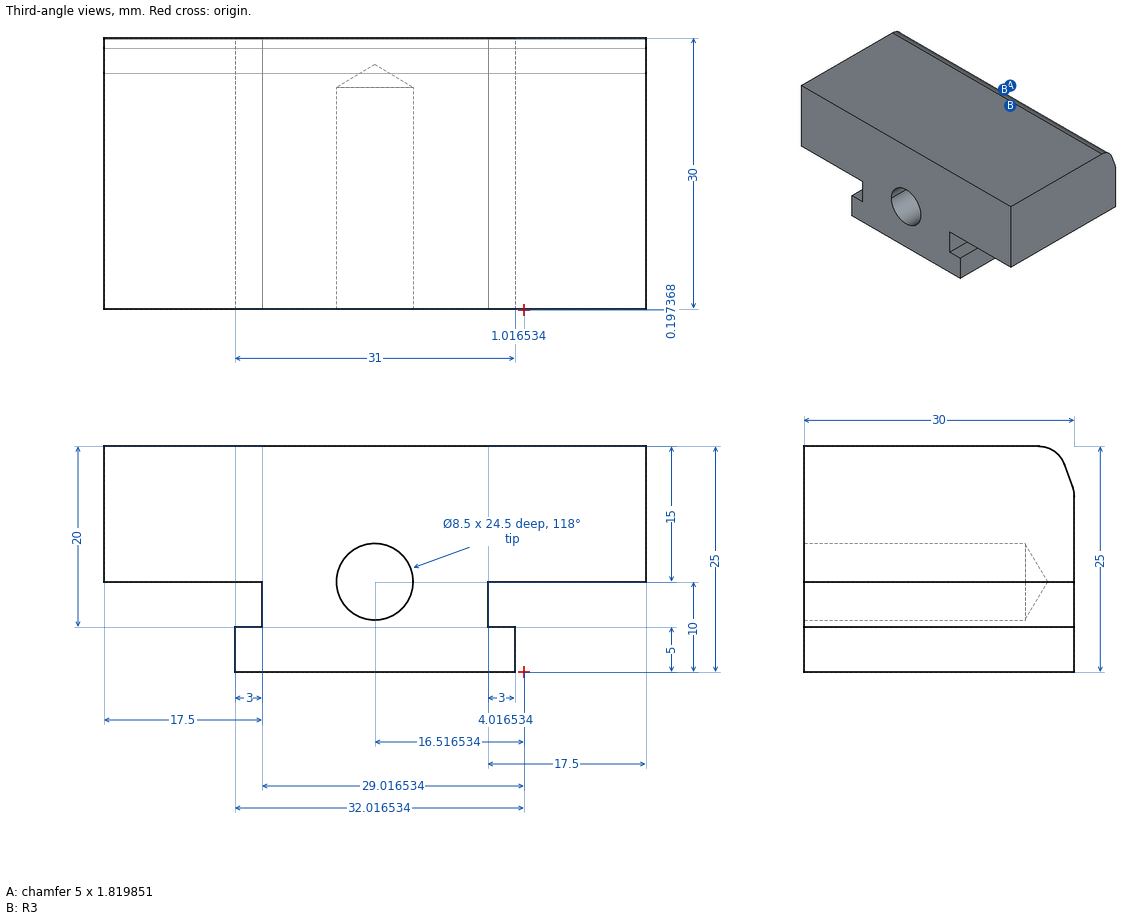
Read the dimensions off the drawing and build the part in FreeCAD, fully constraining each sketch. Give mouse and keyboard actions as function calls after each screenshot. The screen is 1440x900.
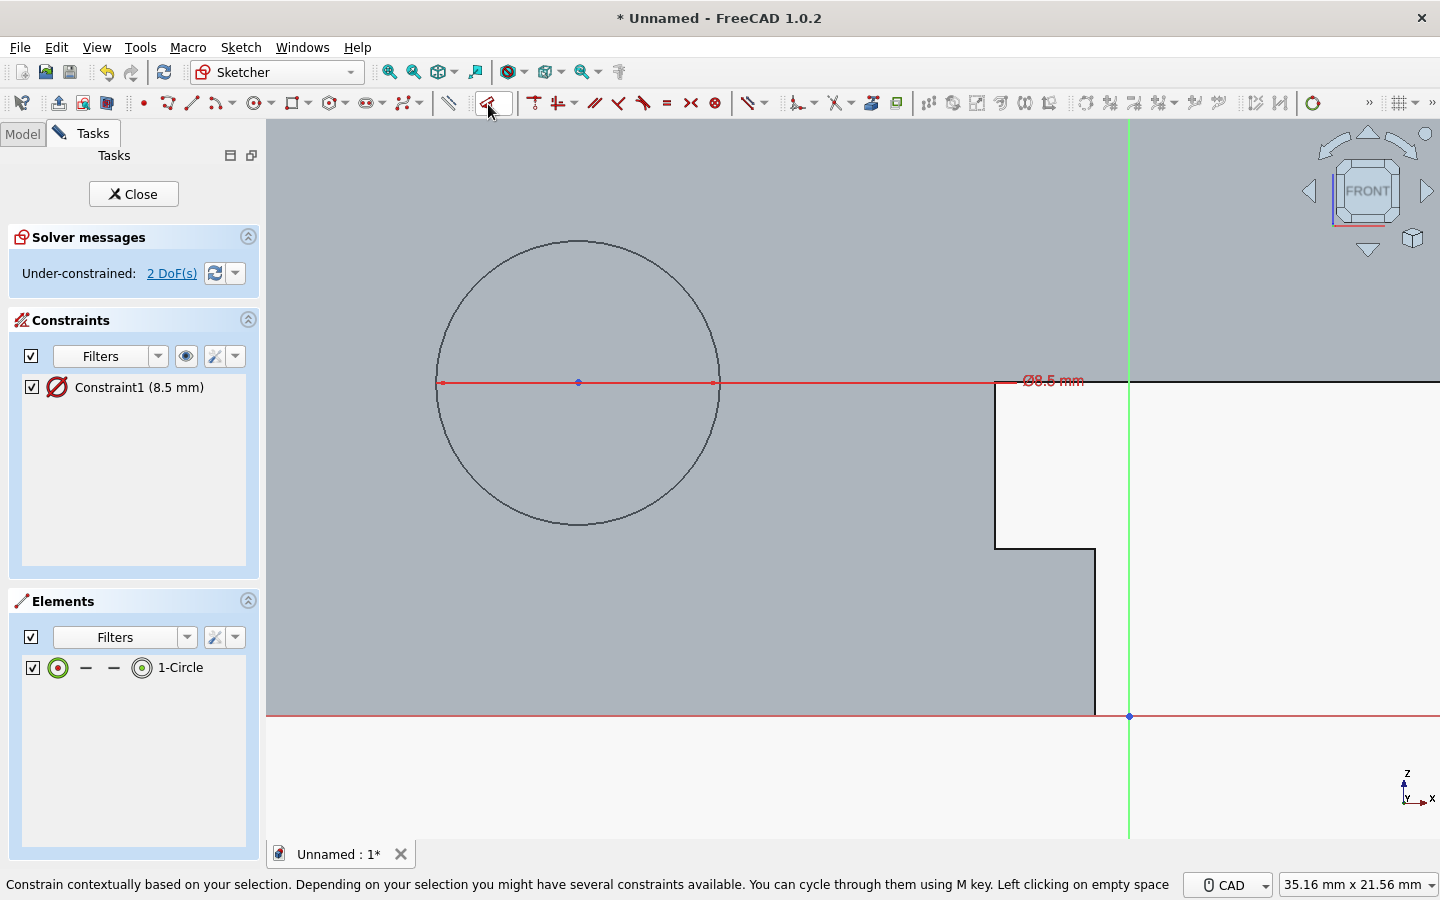
click(578, 383)
click(1163, 550)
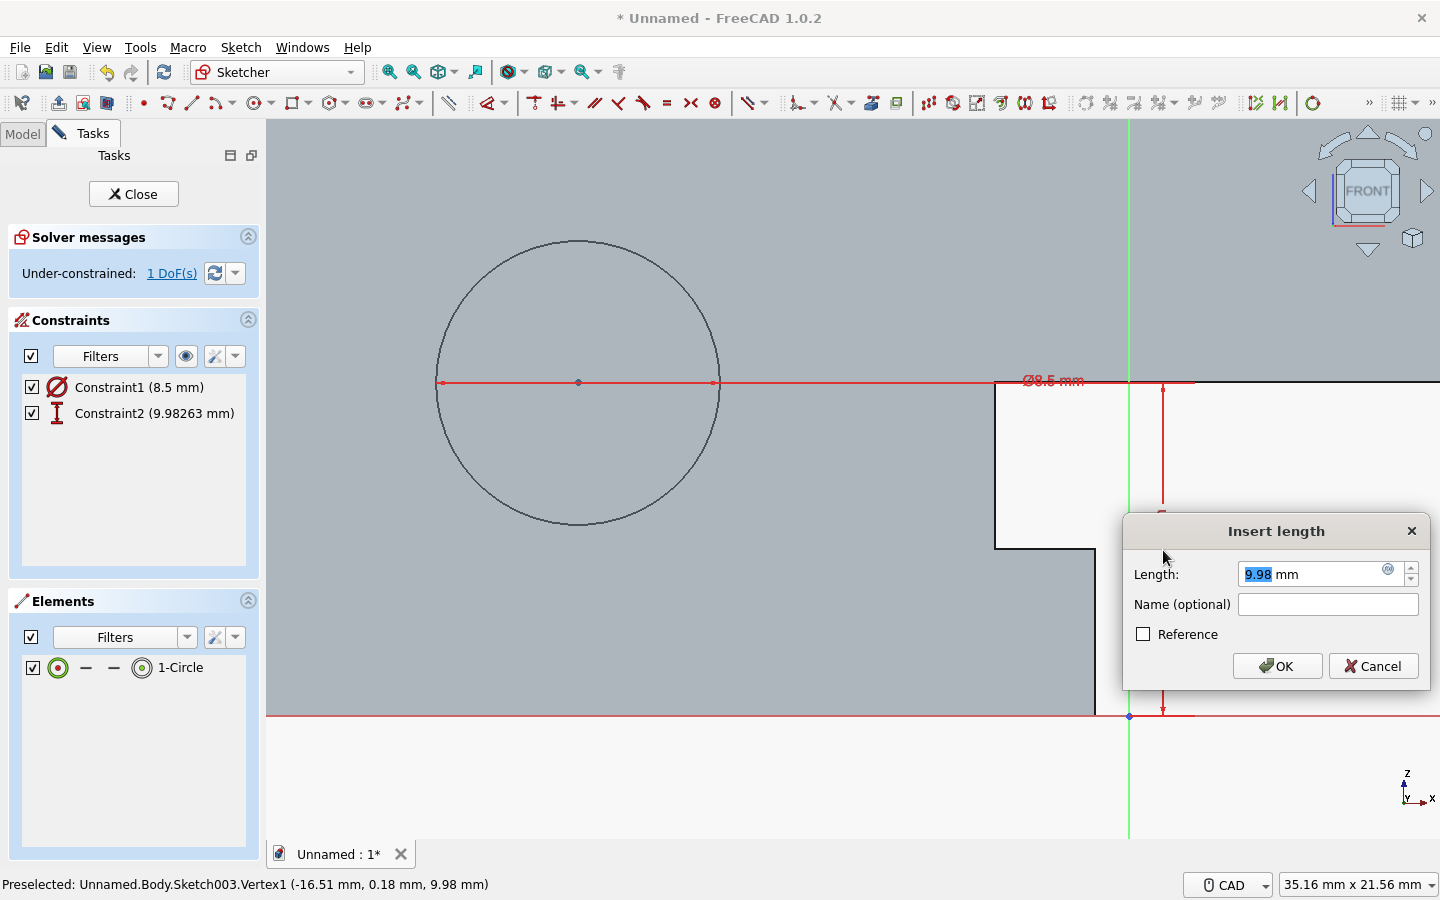
text(10)
key(Return)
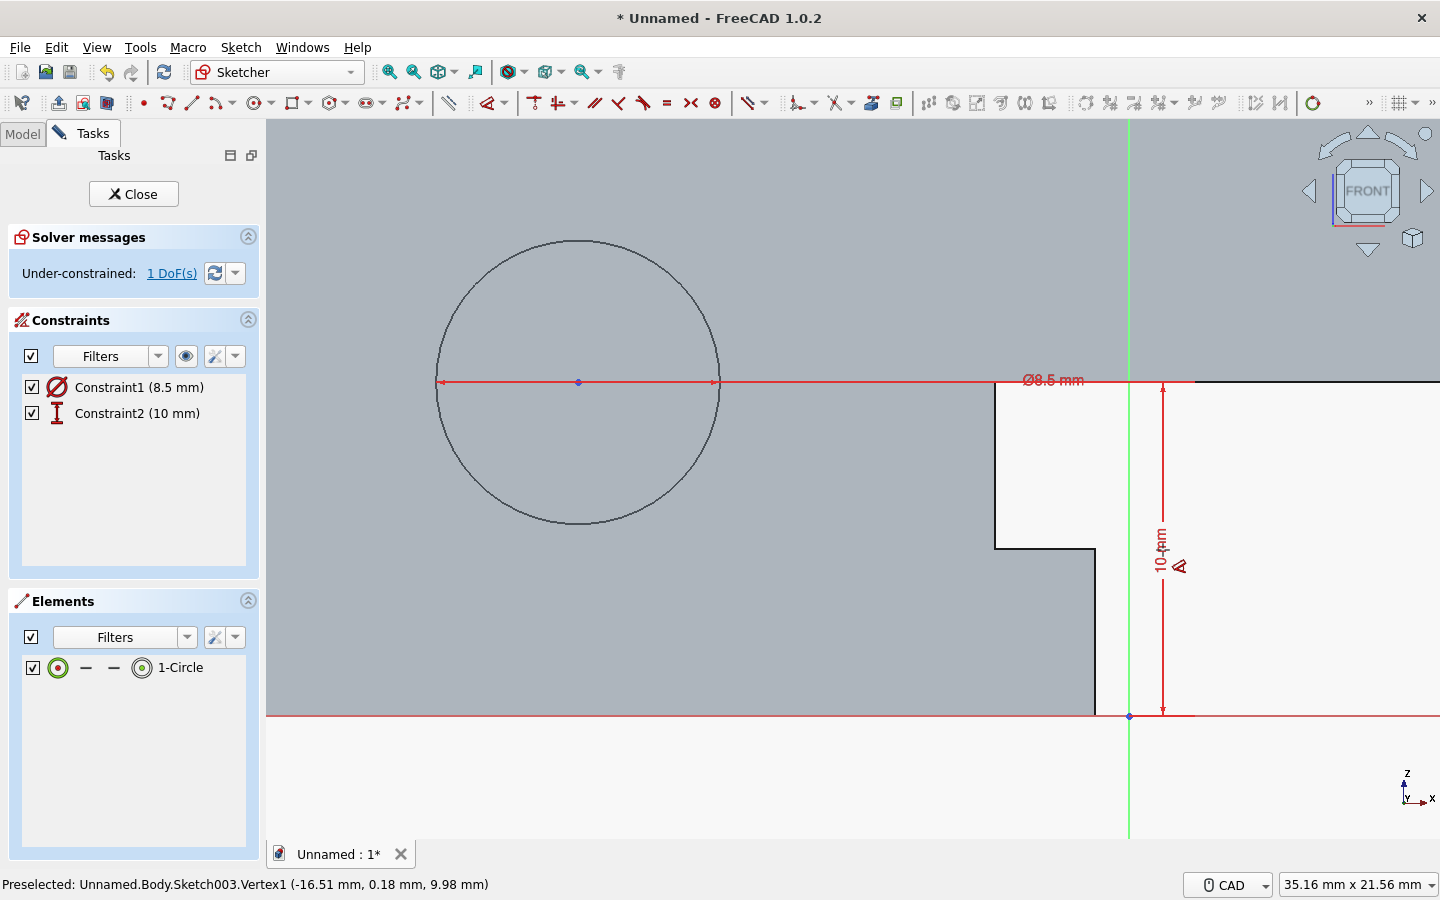
click(578, 382)
click(854, 750)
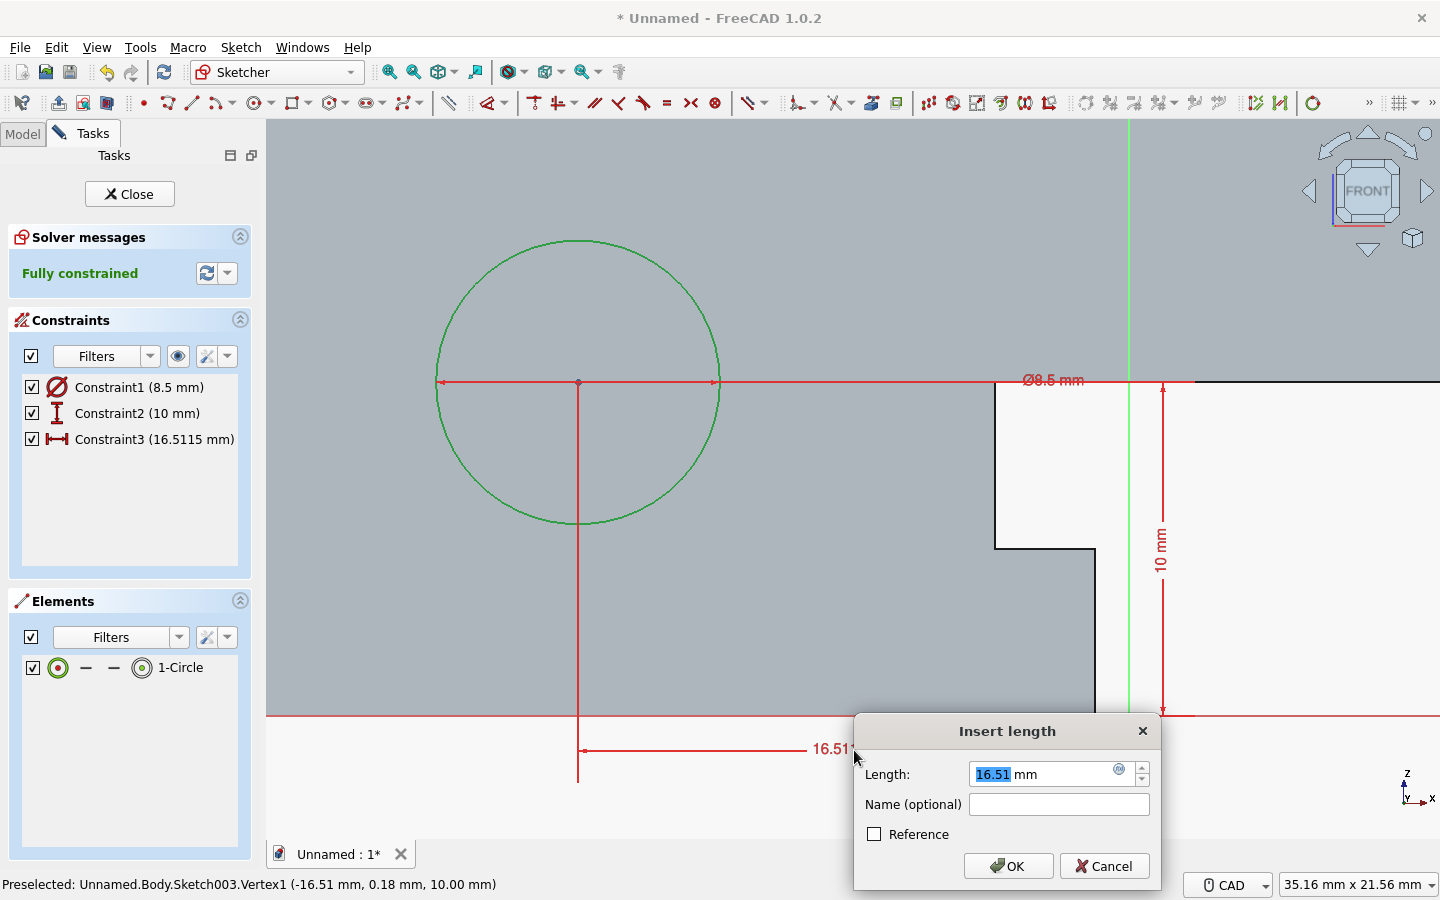
text(16.516534)
key(Return)
key(Escape)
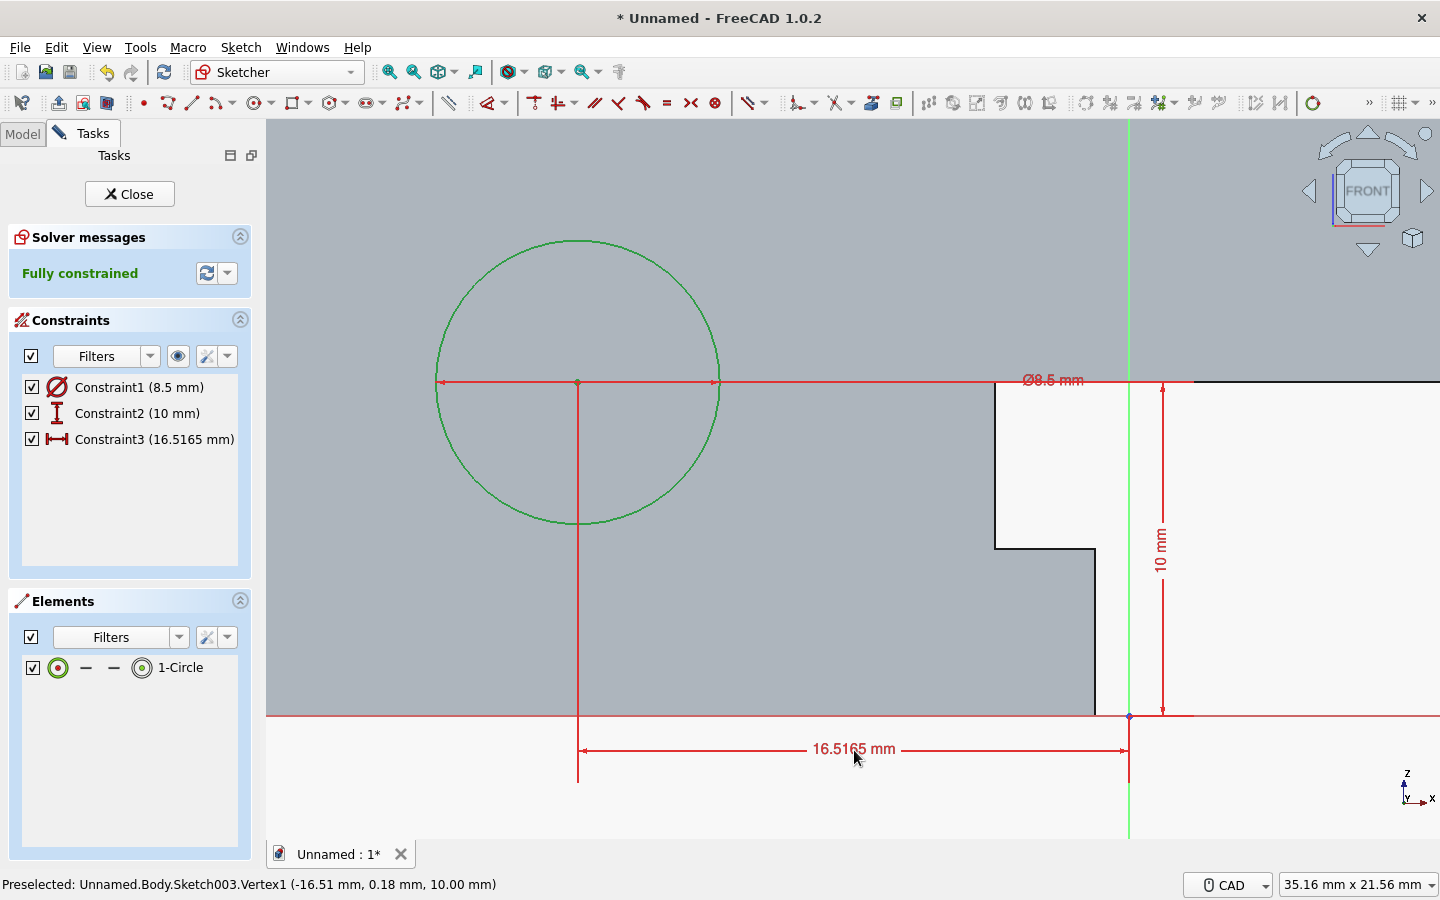
click(130, 194)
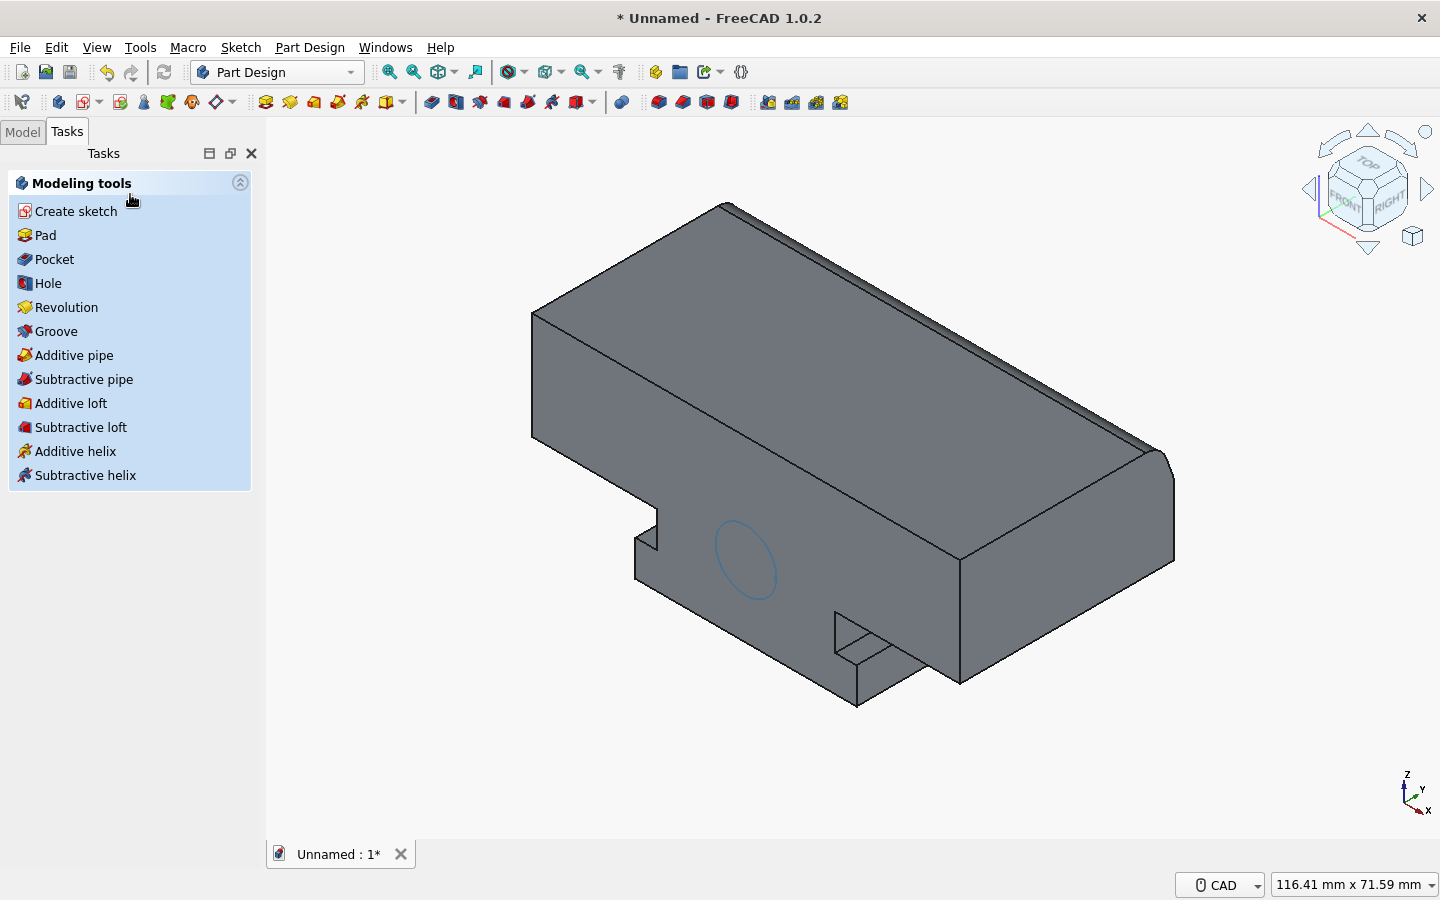
click(456, 102)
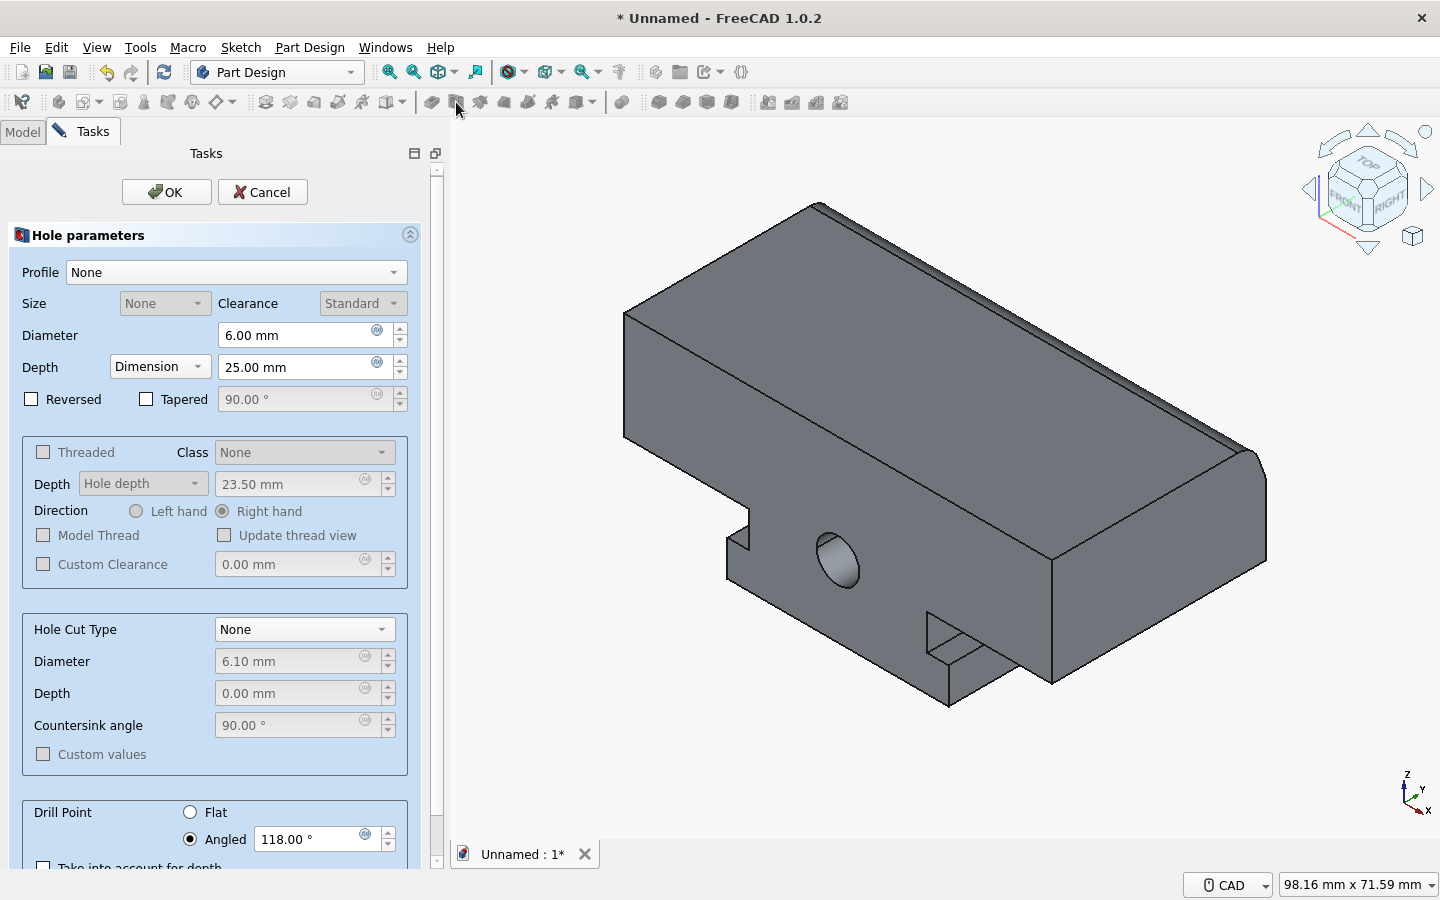
triple_click(305, 335)